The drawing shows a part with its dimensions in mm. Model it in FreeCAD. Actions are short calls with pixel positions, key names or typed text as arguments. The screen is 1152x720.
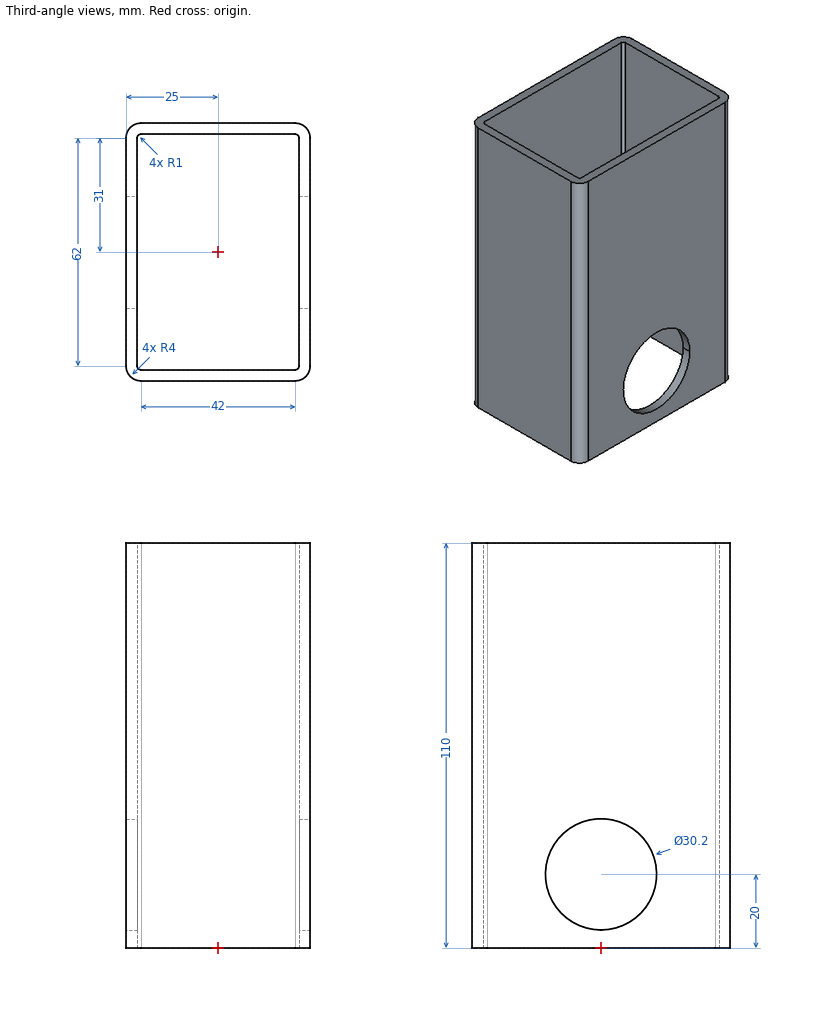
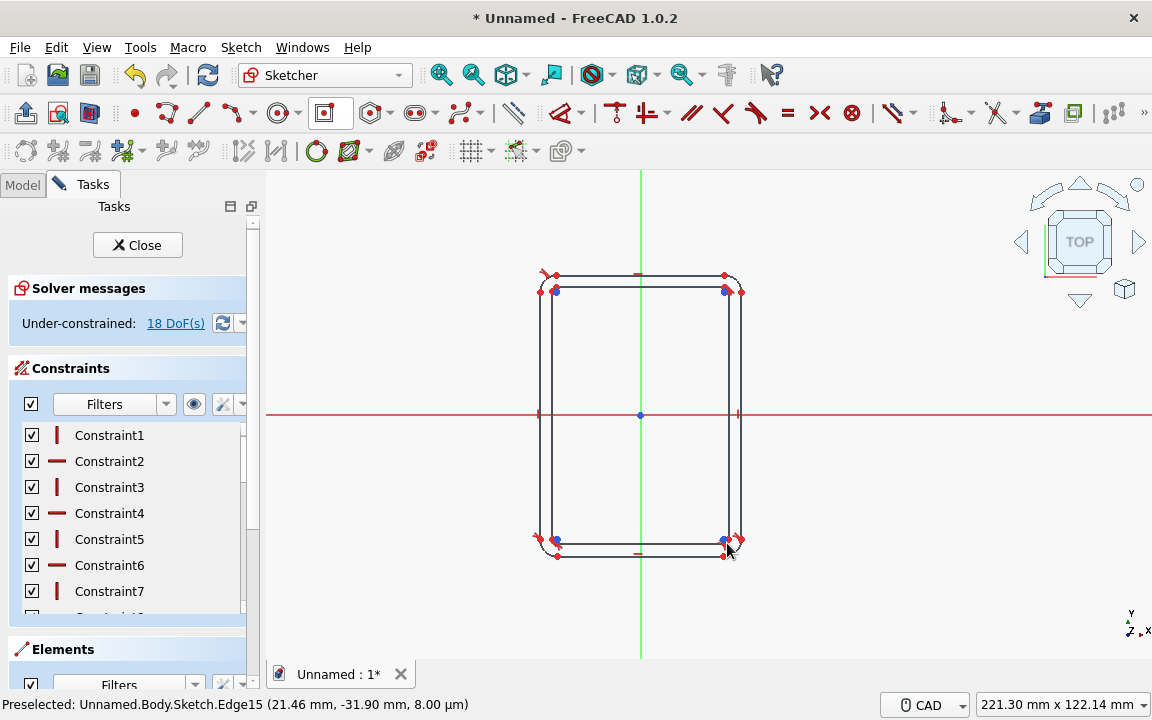
click(674, 544)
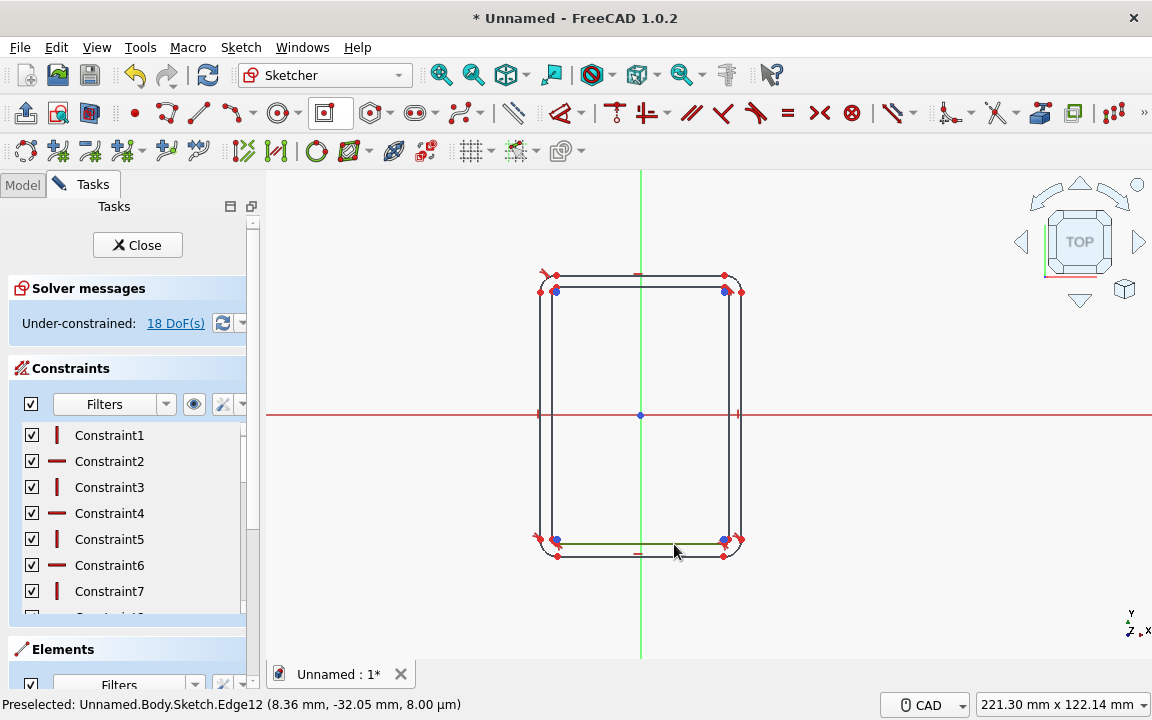
scroll(727, 542, up, 8)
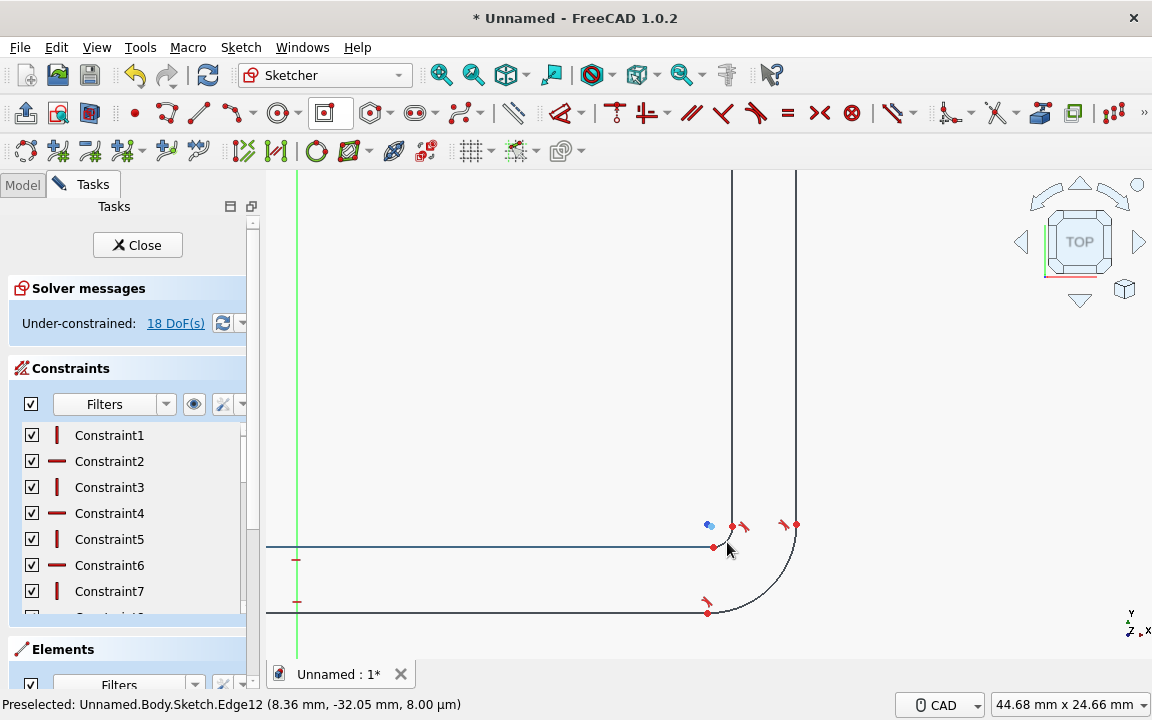
click(727, 541)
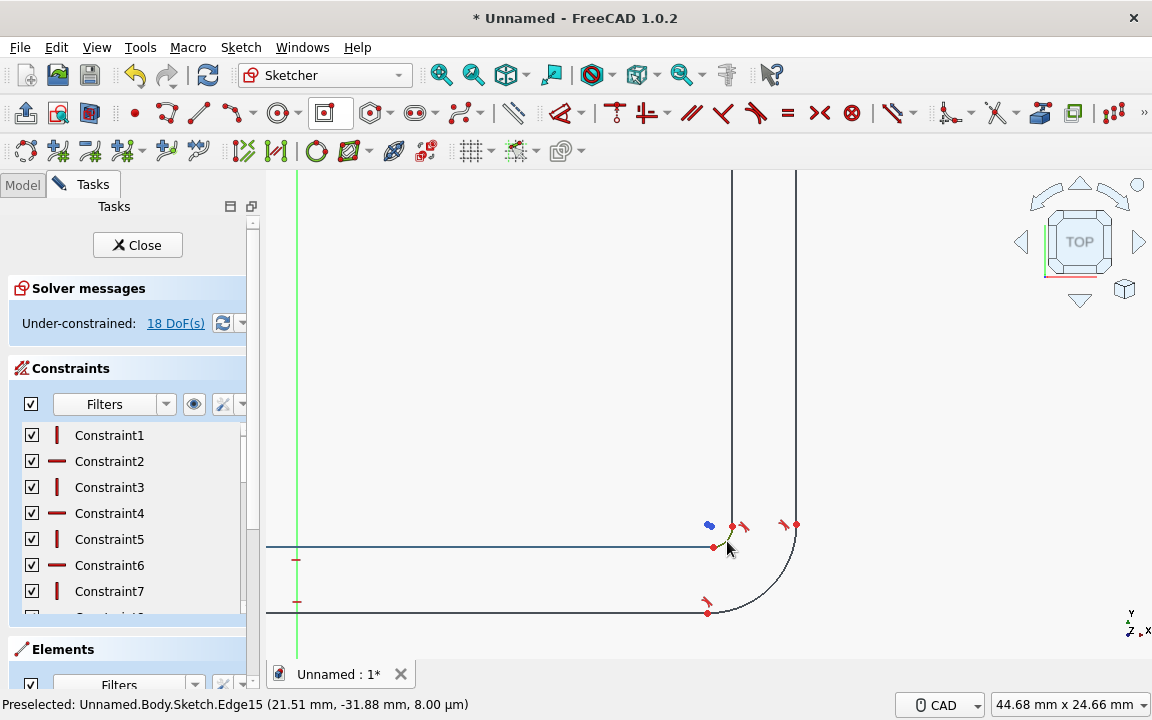
key(t)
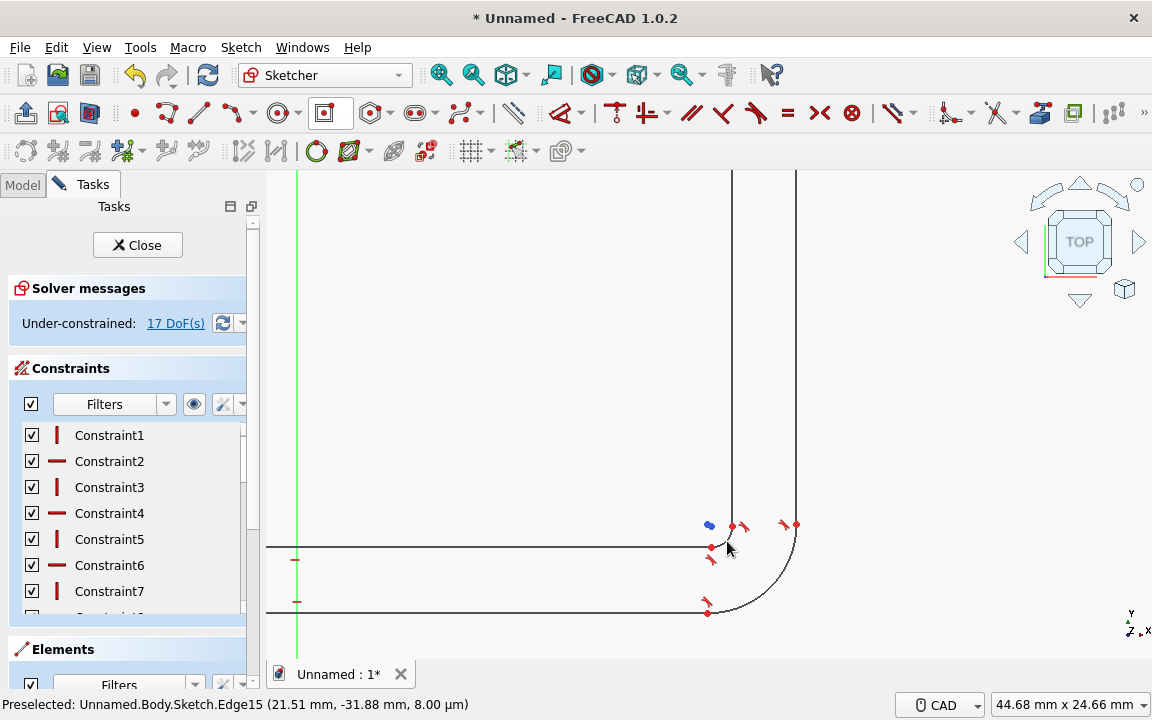
scroll(727, 542, down, 8)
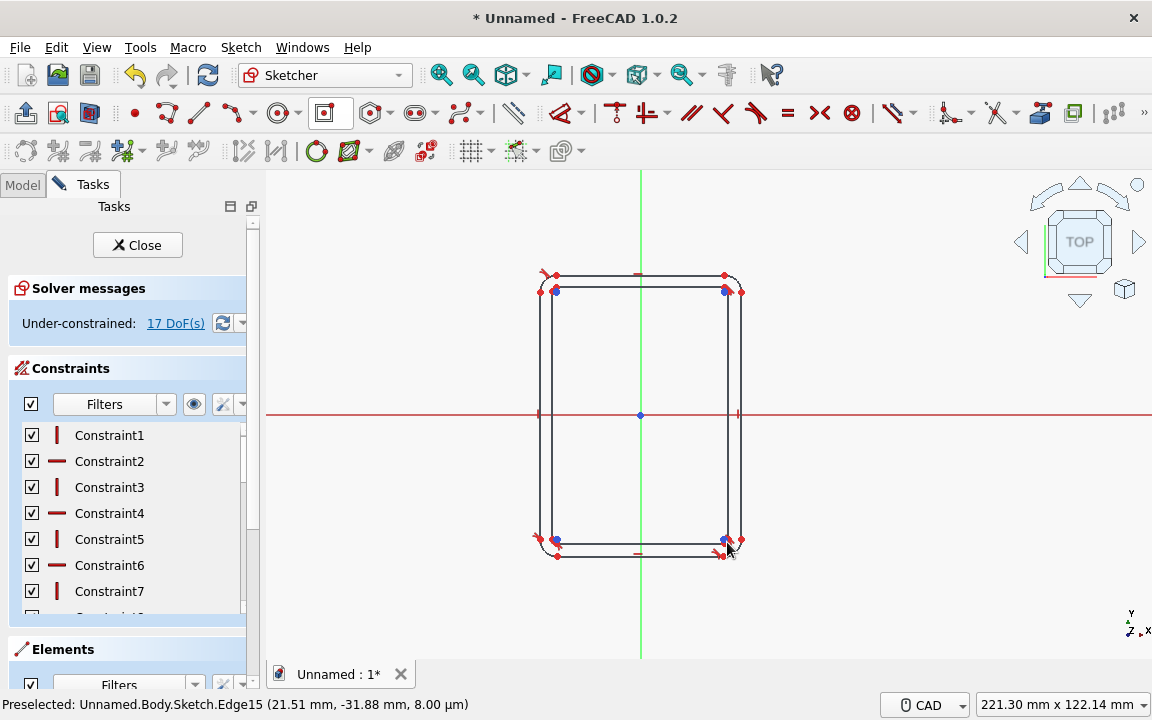
click(674, 544)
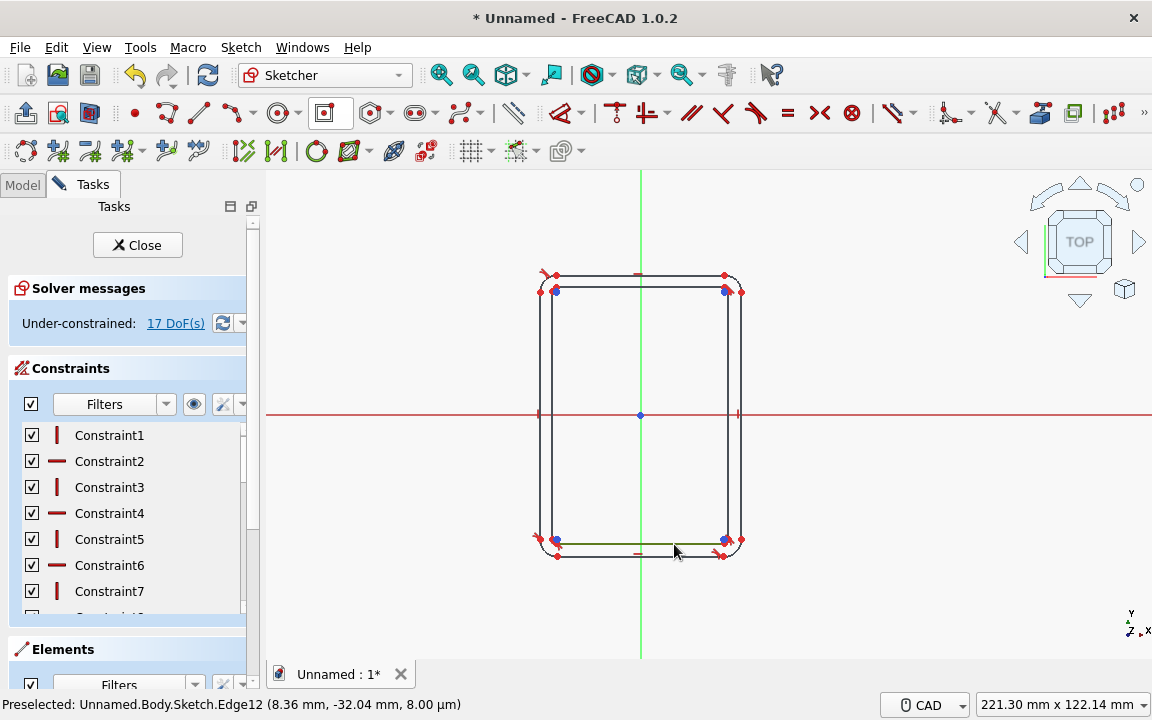
scroll(554, 542, up, 8)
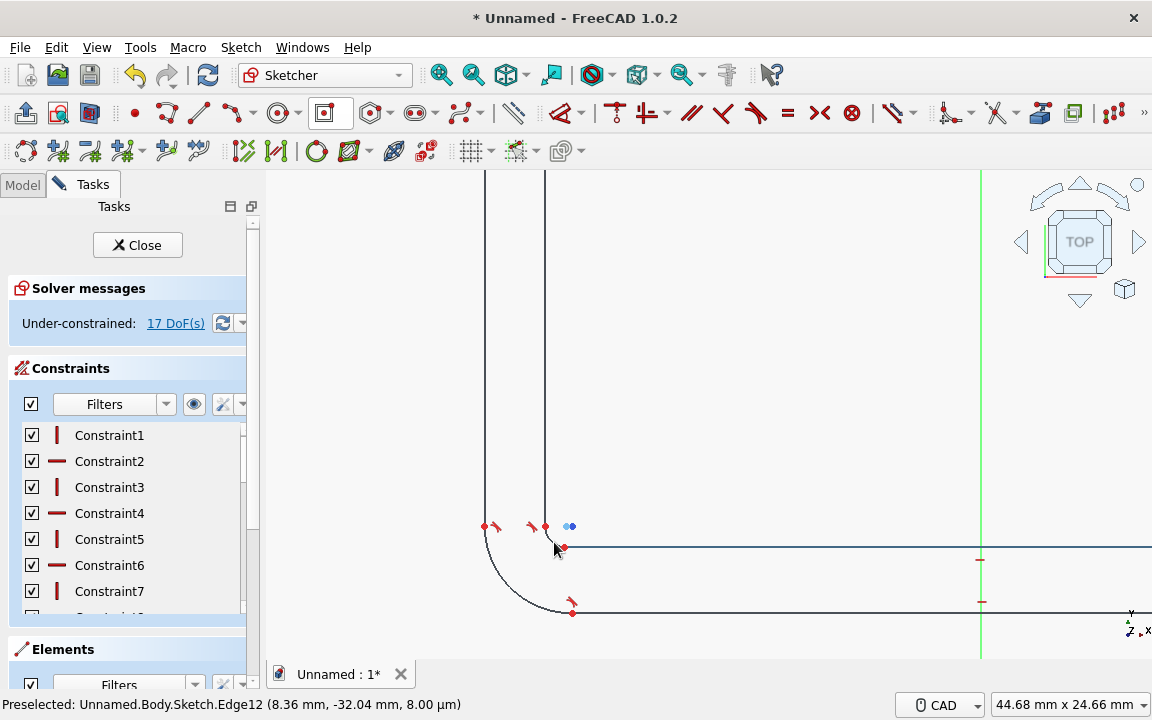
click(551, 541)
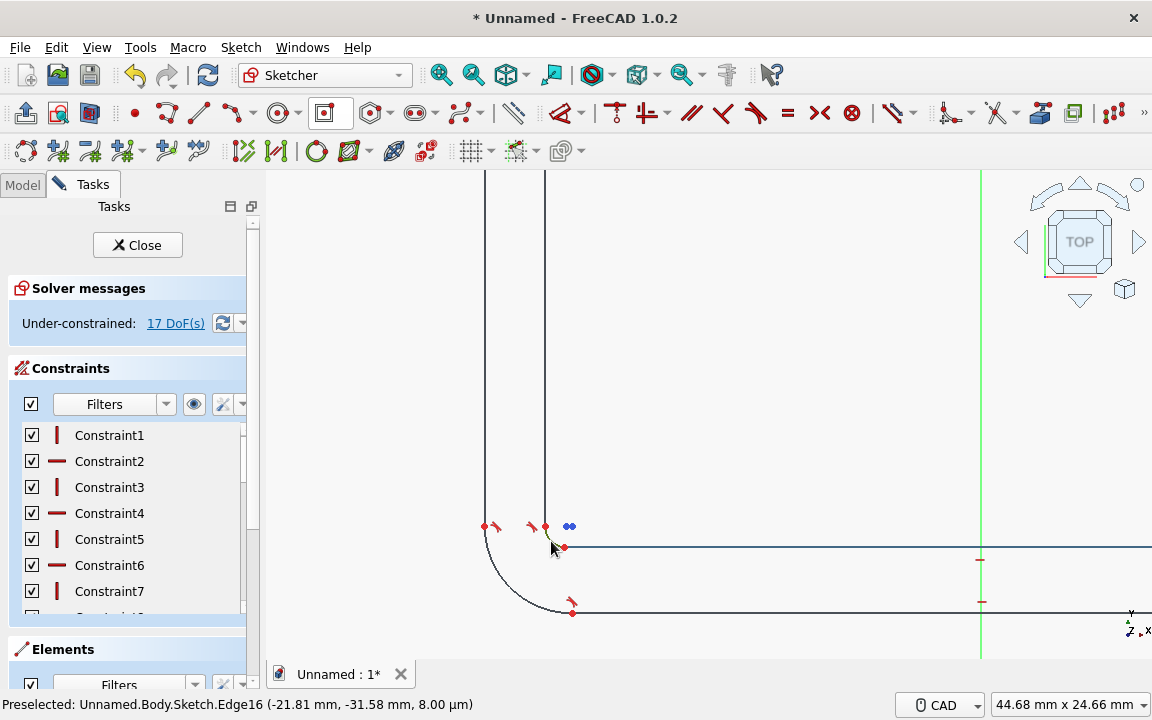
key(t)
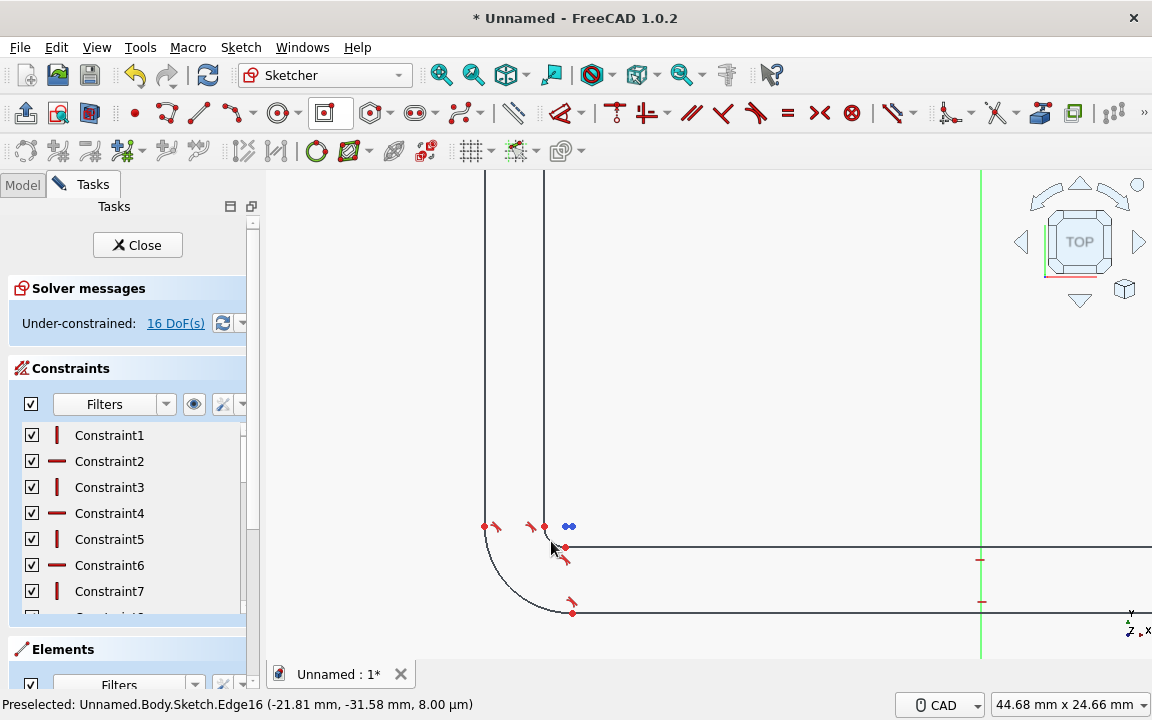
scroll(554, 542, down, 8)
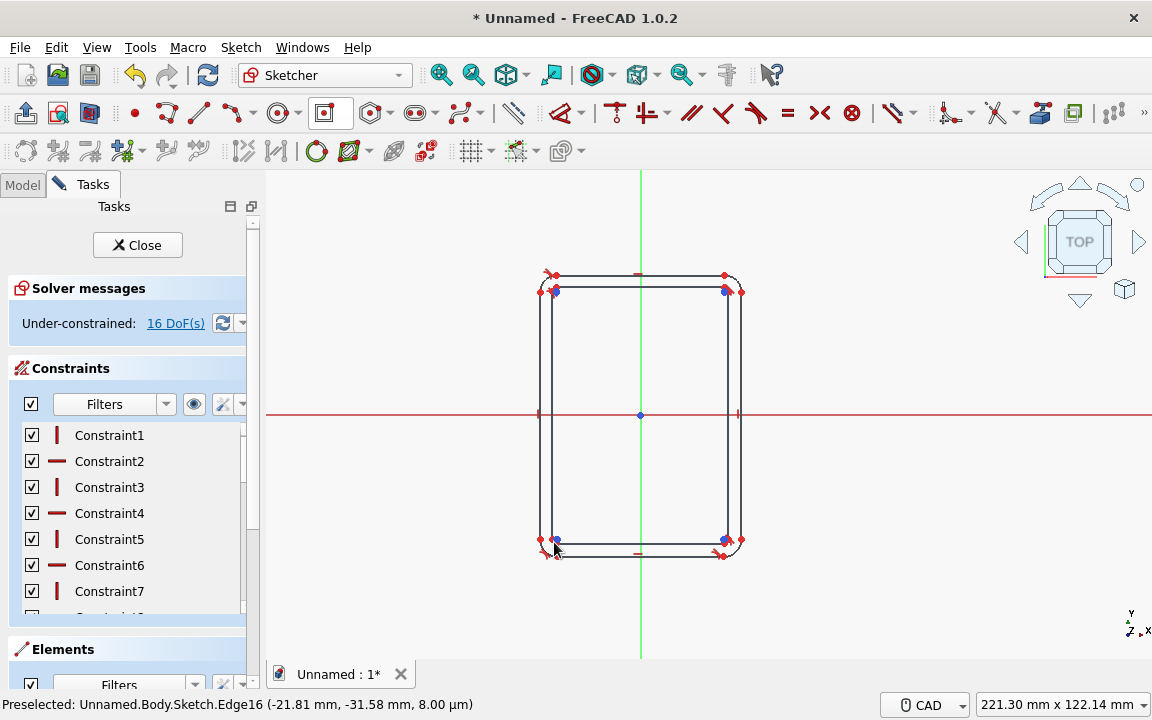
scroll(549, 277, up, 3)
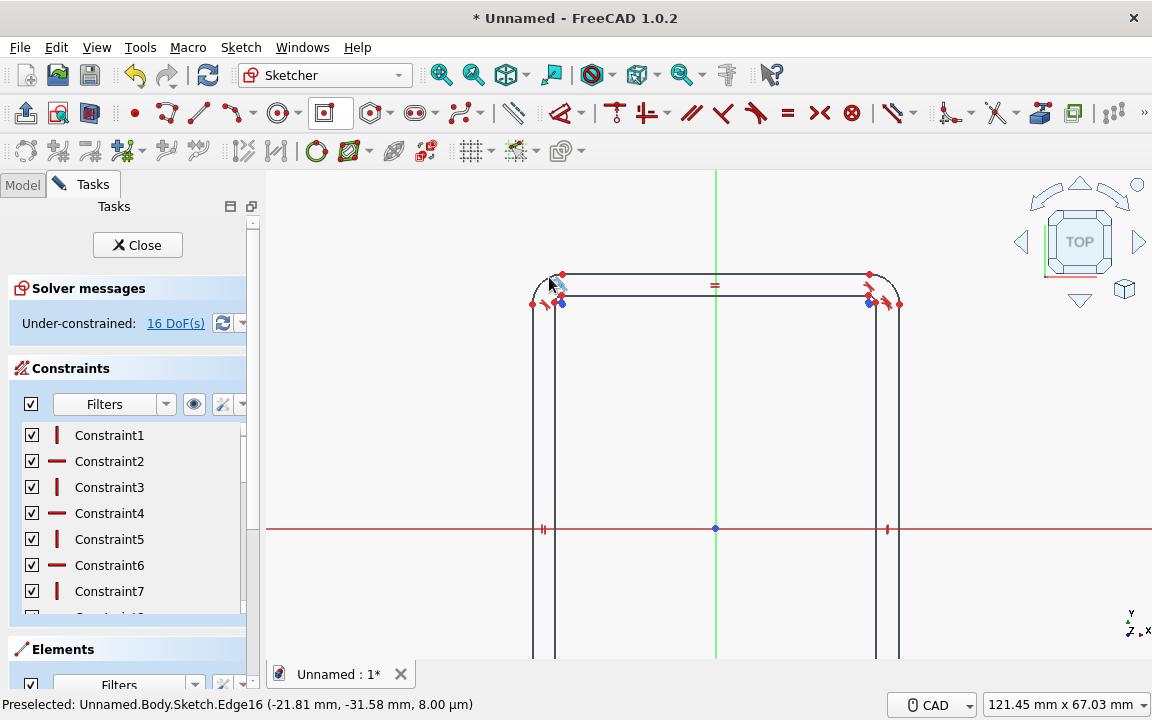
click(549, 278)